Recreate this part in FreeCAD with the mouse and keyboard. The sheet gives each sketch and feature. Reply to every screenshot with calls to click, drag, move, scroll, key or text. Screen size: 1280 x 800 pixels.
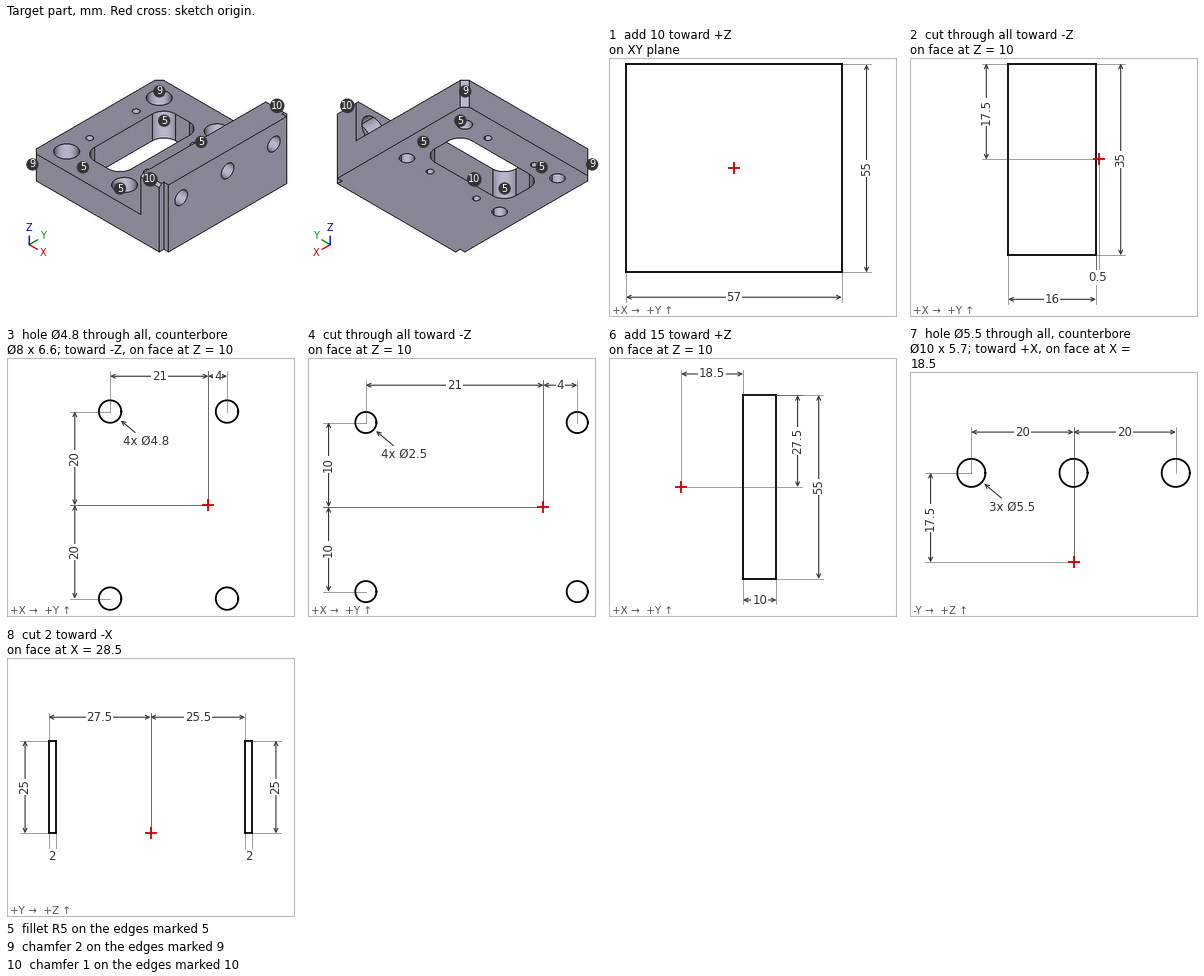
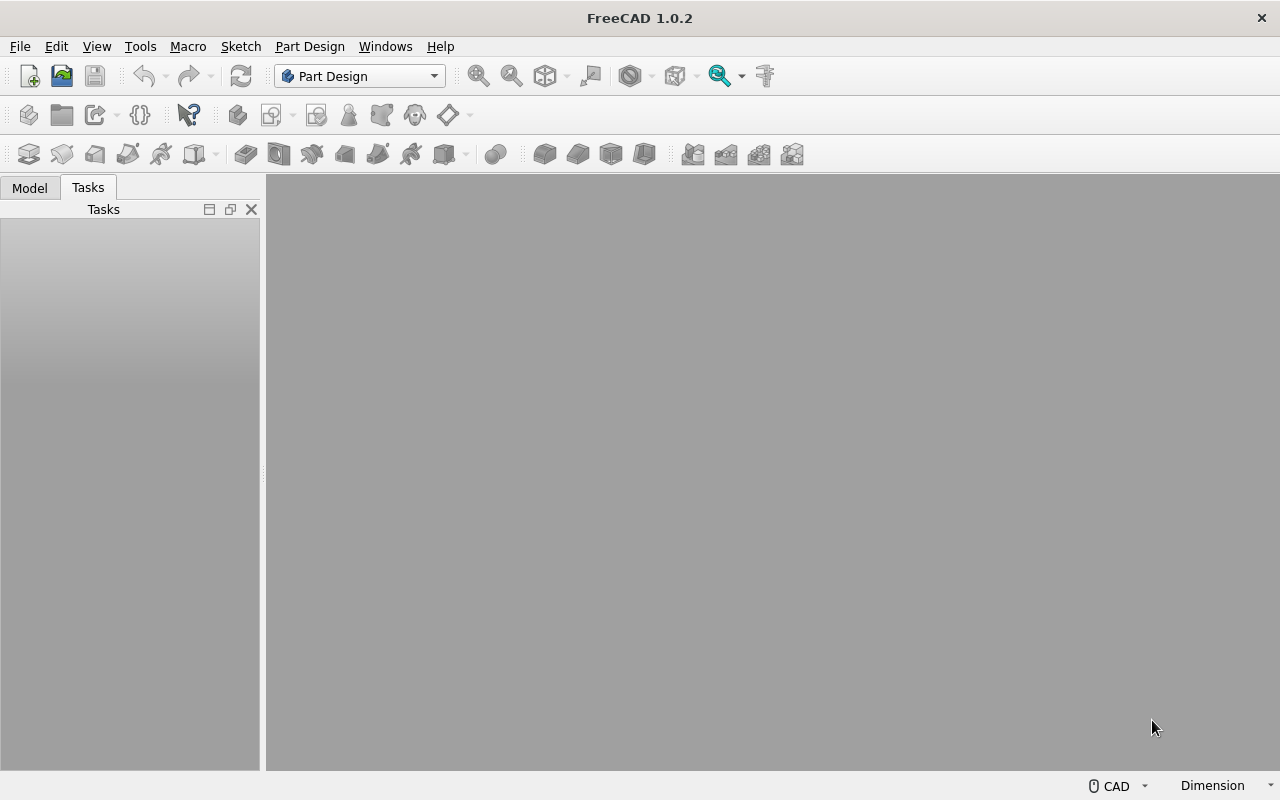
click(29, 76)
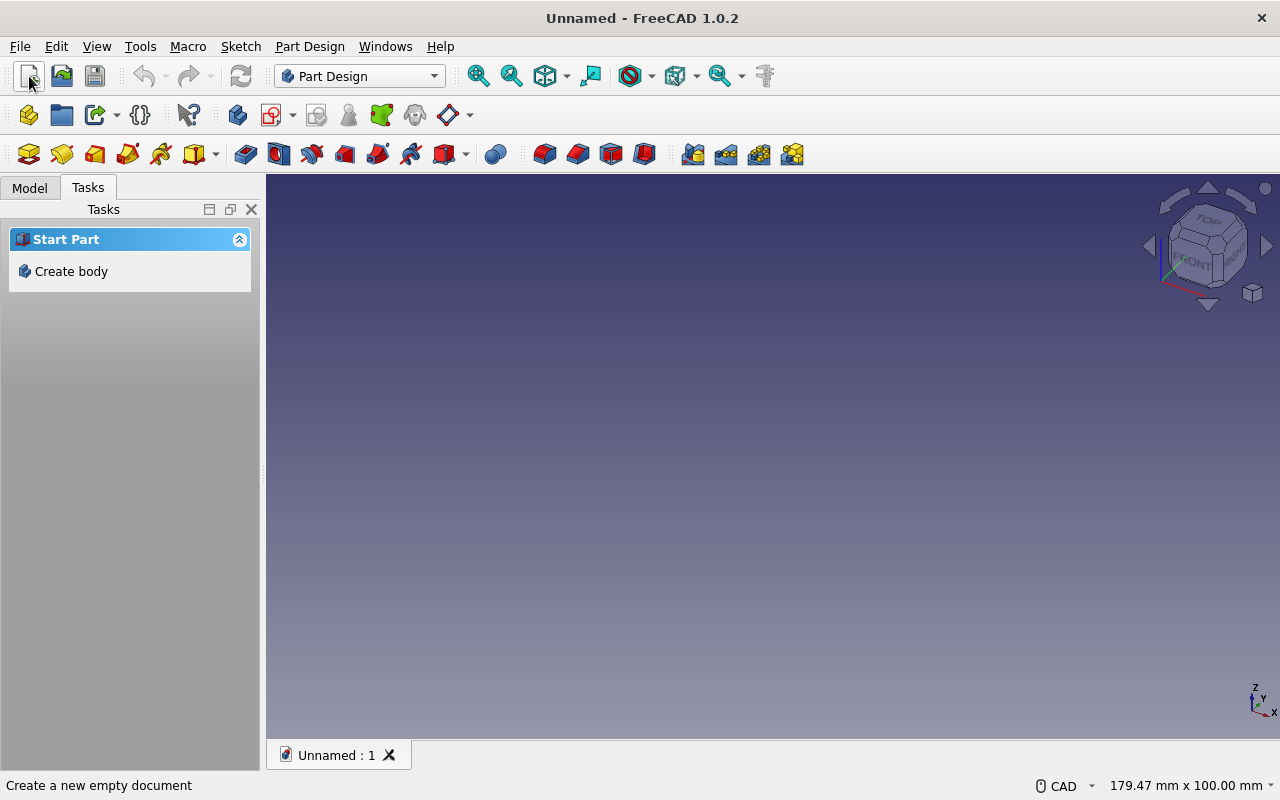
click(270, 116)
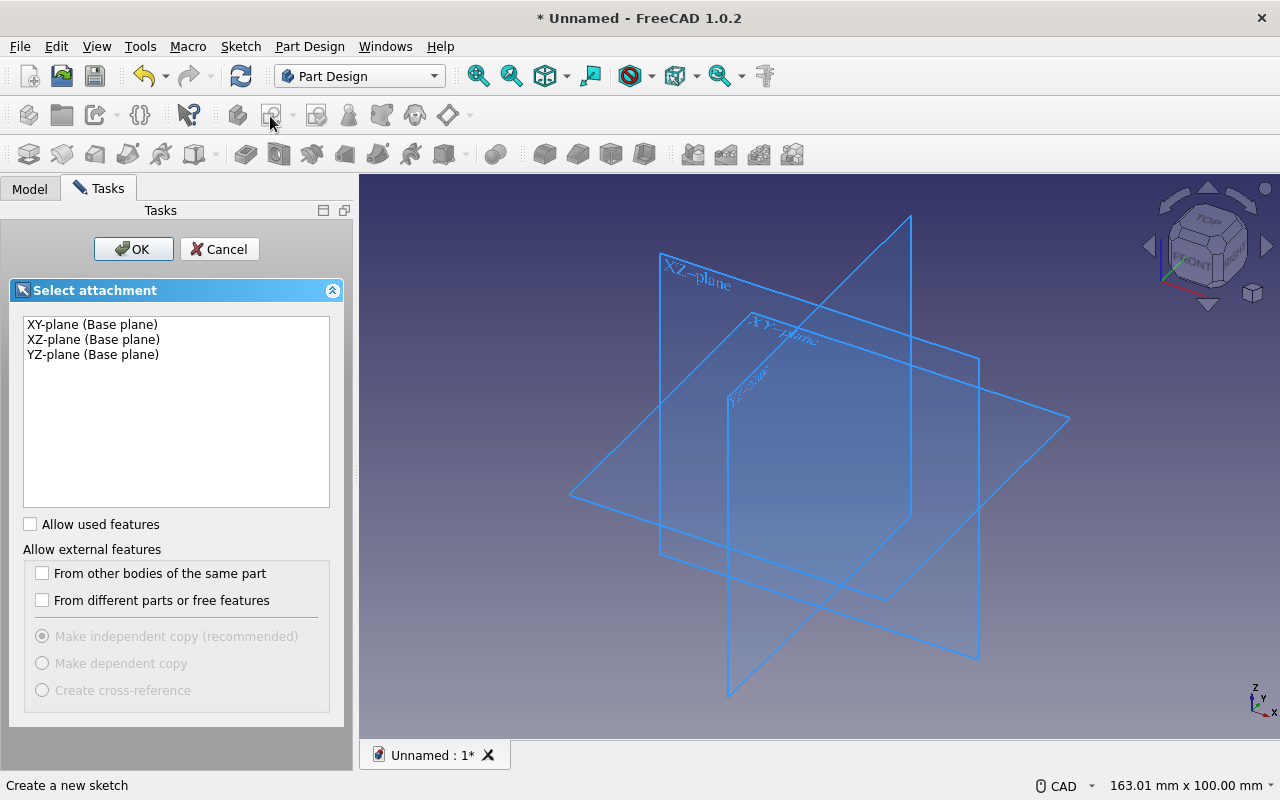
click(84, 324)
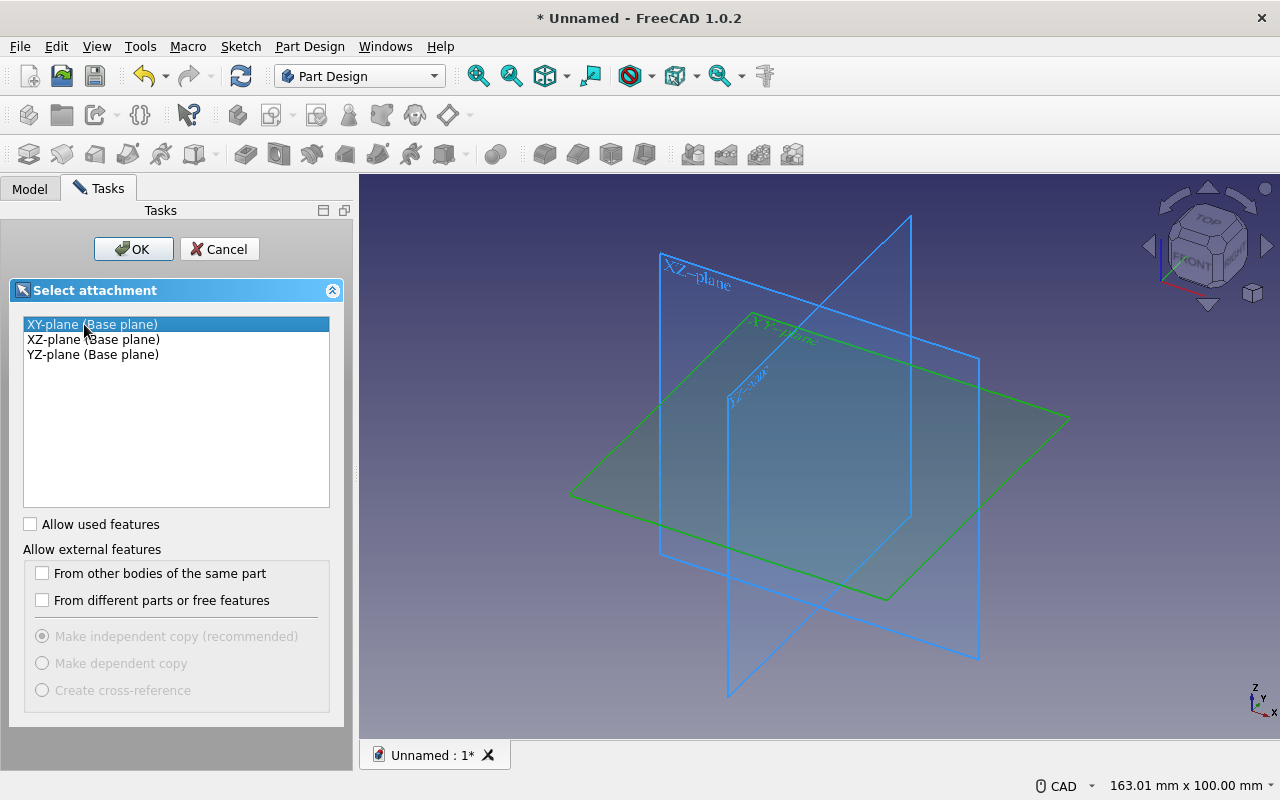
click(134, 249)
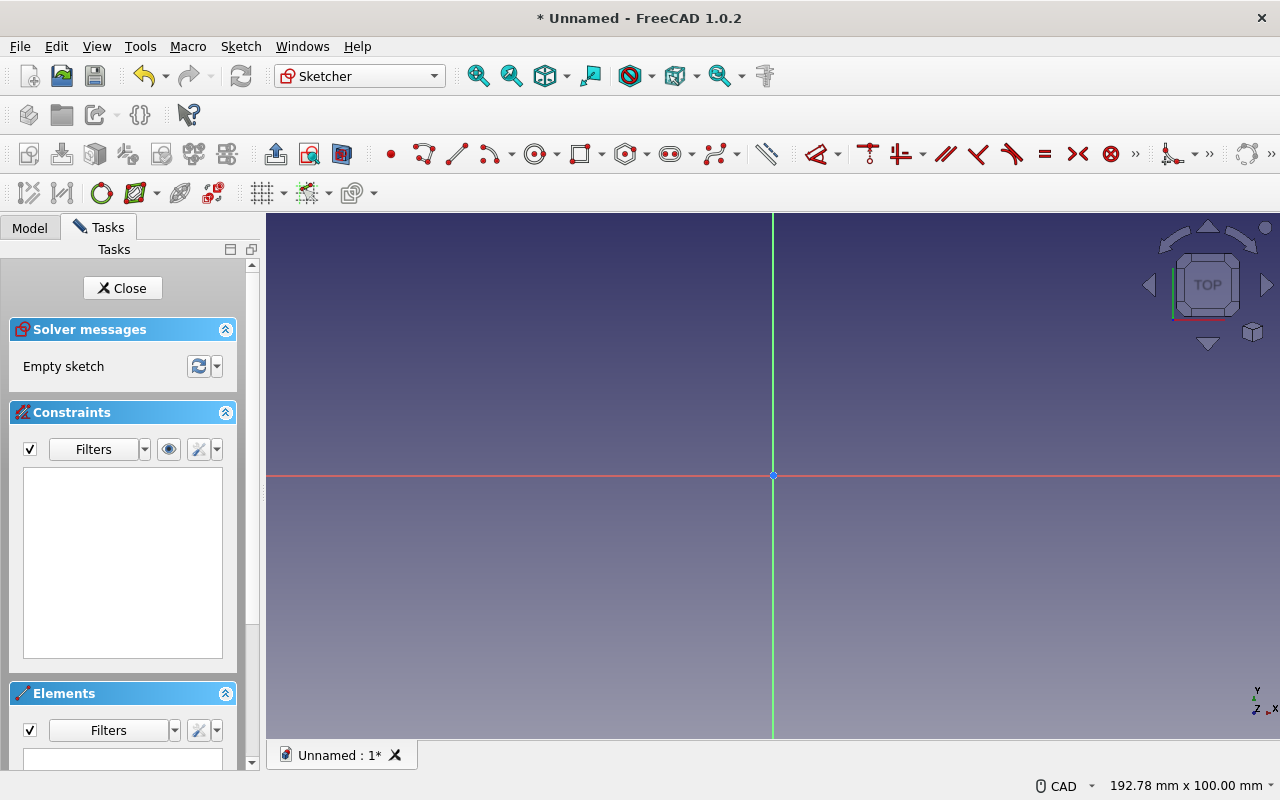
click(602, 154)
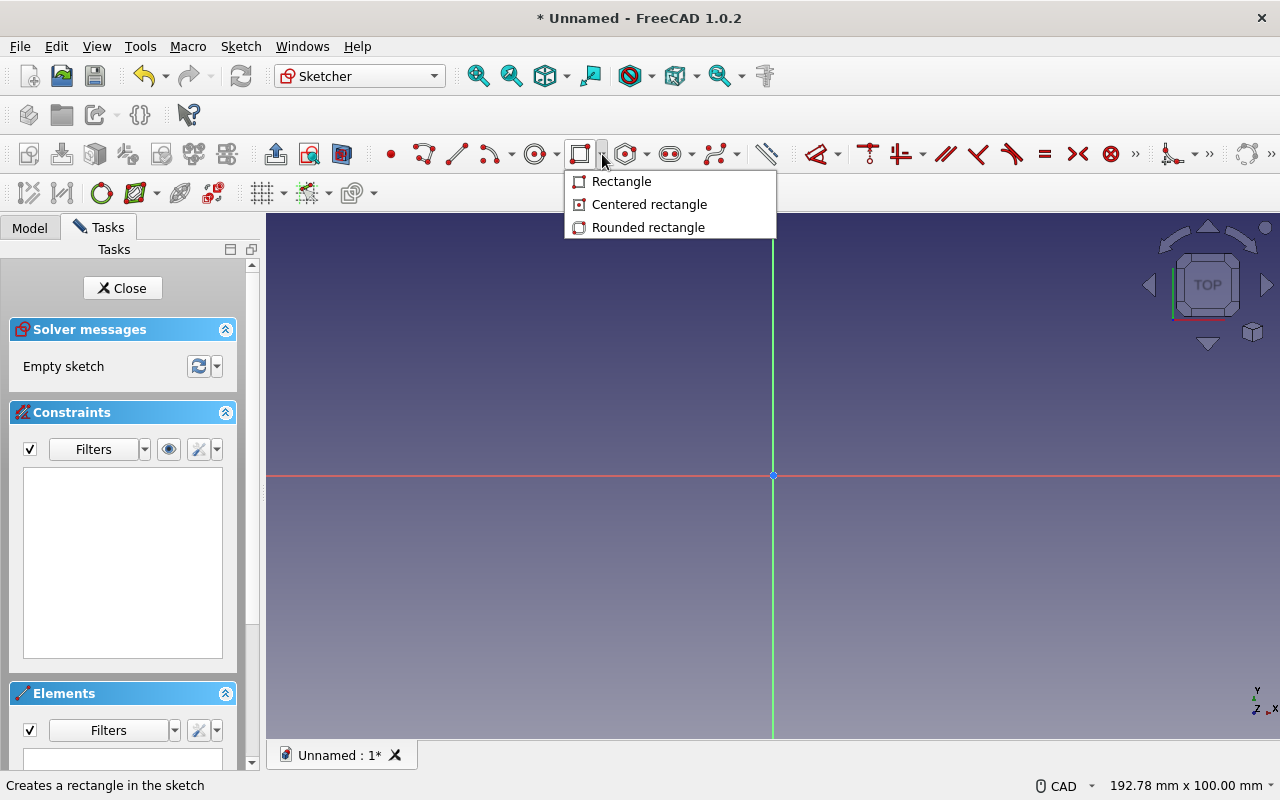
click(670, 204)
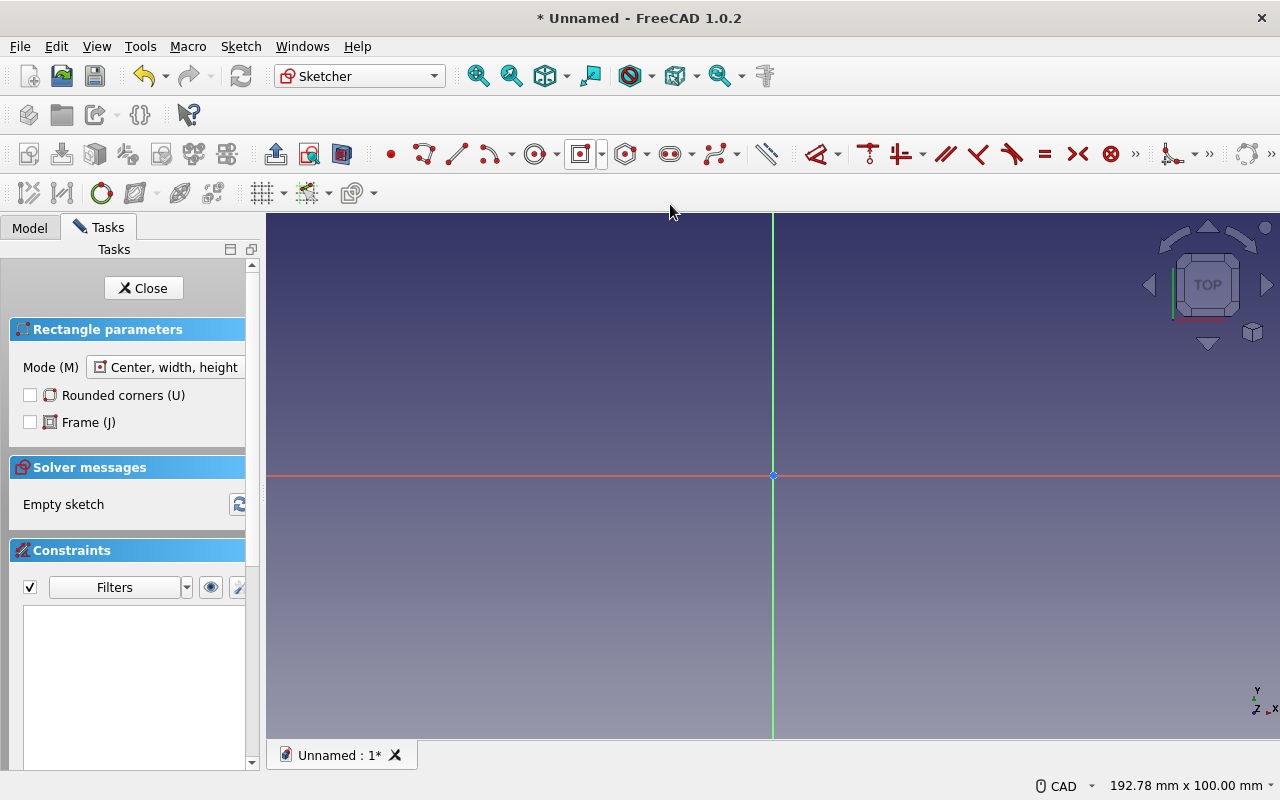
click(773, 476)
move(923, 331)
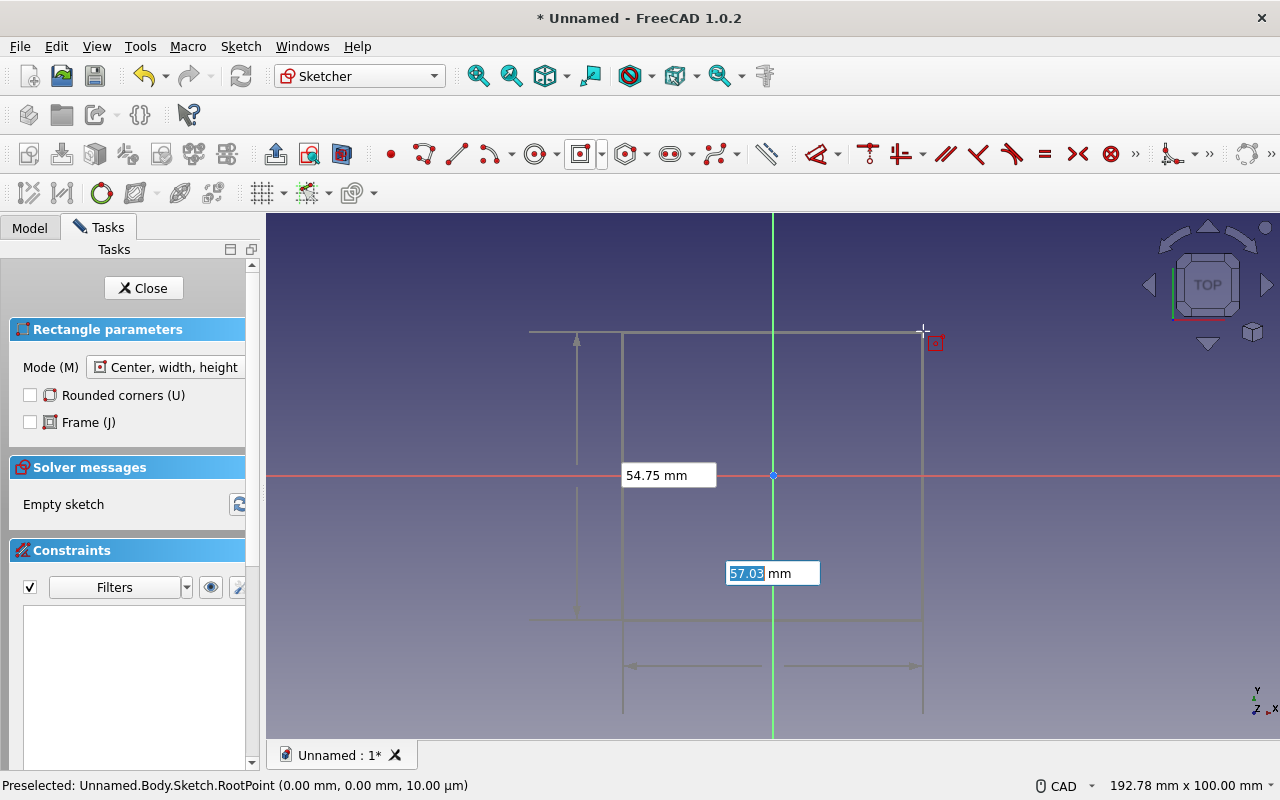
text(57)
key(Tab)
text(55)
key(Return)
key(Escape)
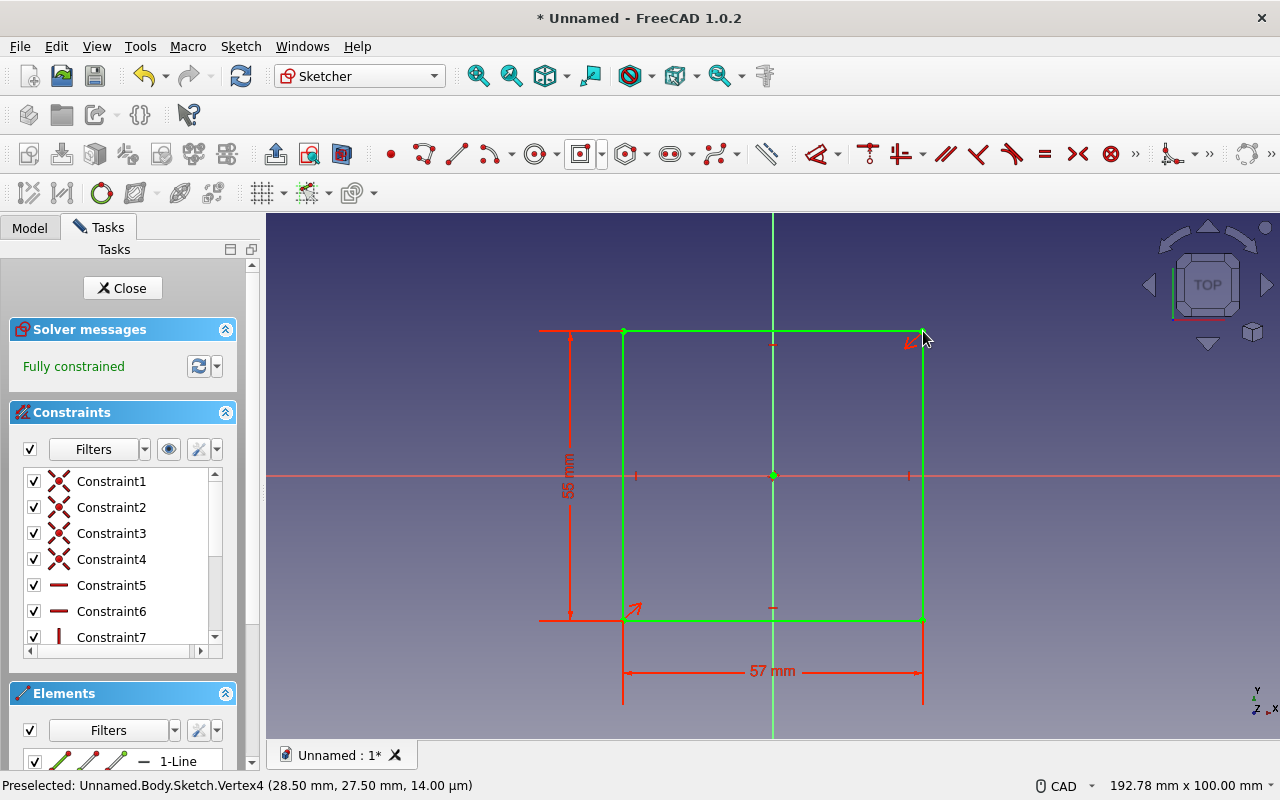
click(123, 288)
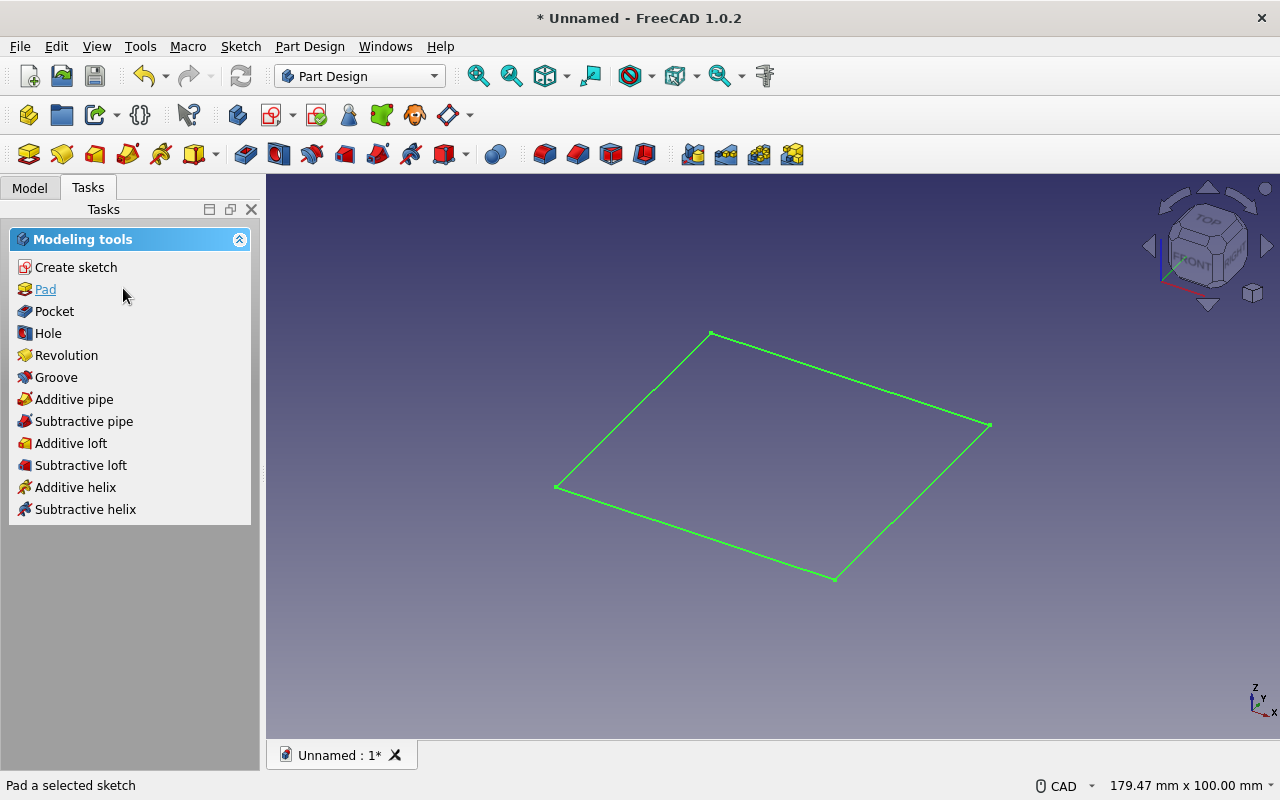
click(29, 154)